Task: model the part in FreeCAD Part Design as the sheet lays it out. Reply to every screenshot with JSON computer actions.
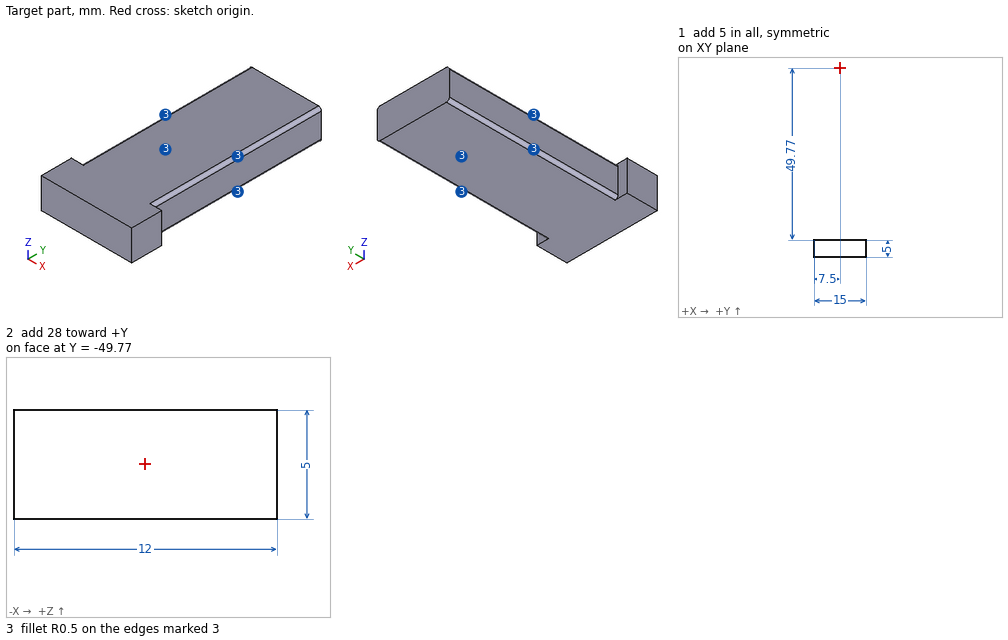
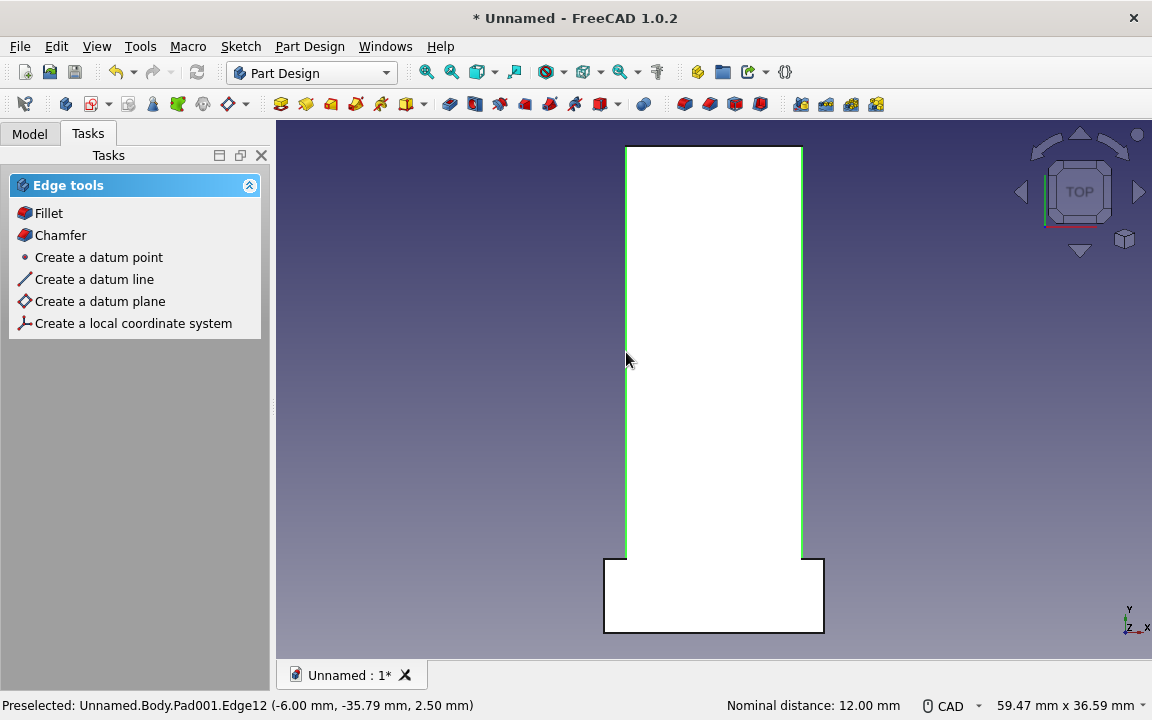
{"action": "left_click", "coordinate": [427, 72]}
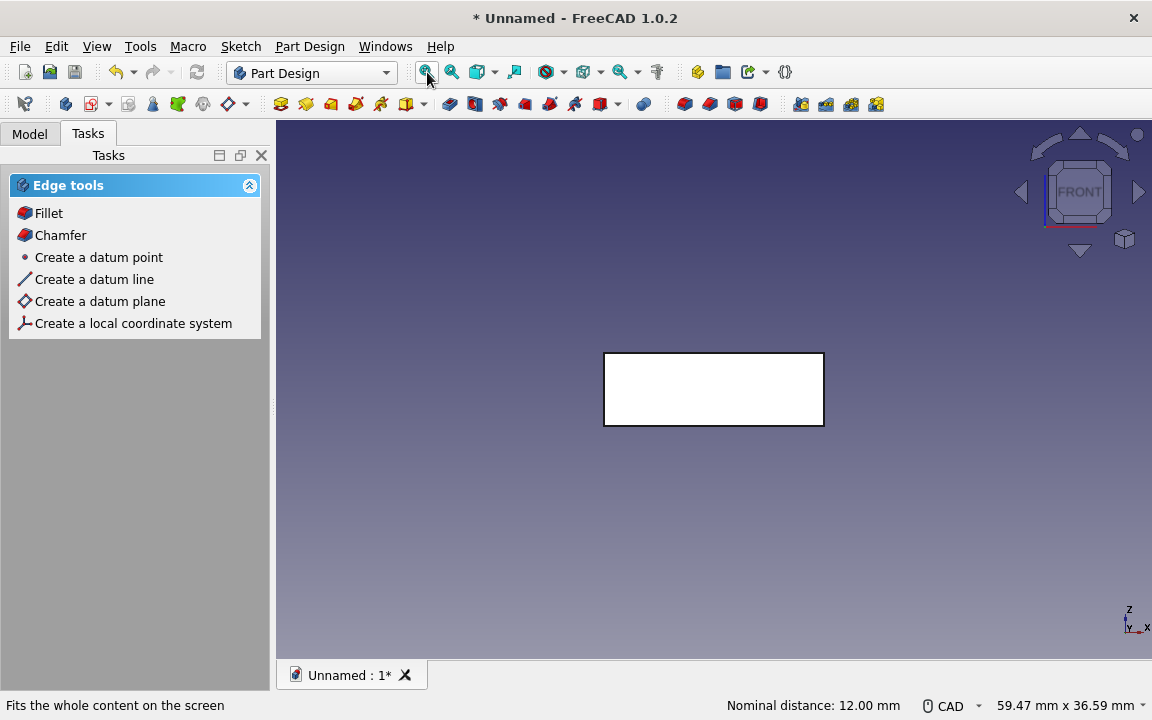
{"action": "key", "text": "3"}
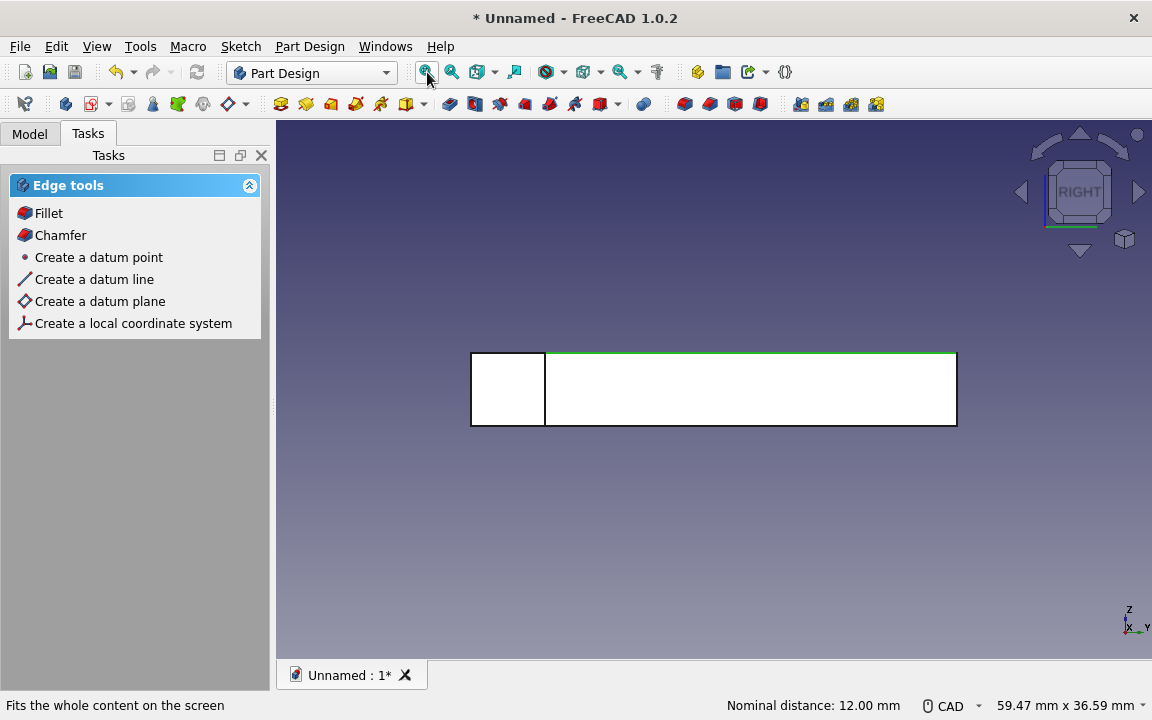
{"action": "left_click", "coordinate": [751, 425], "text": "ctrl"}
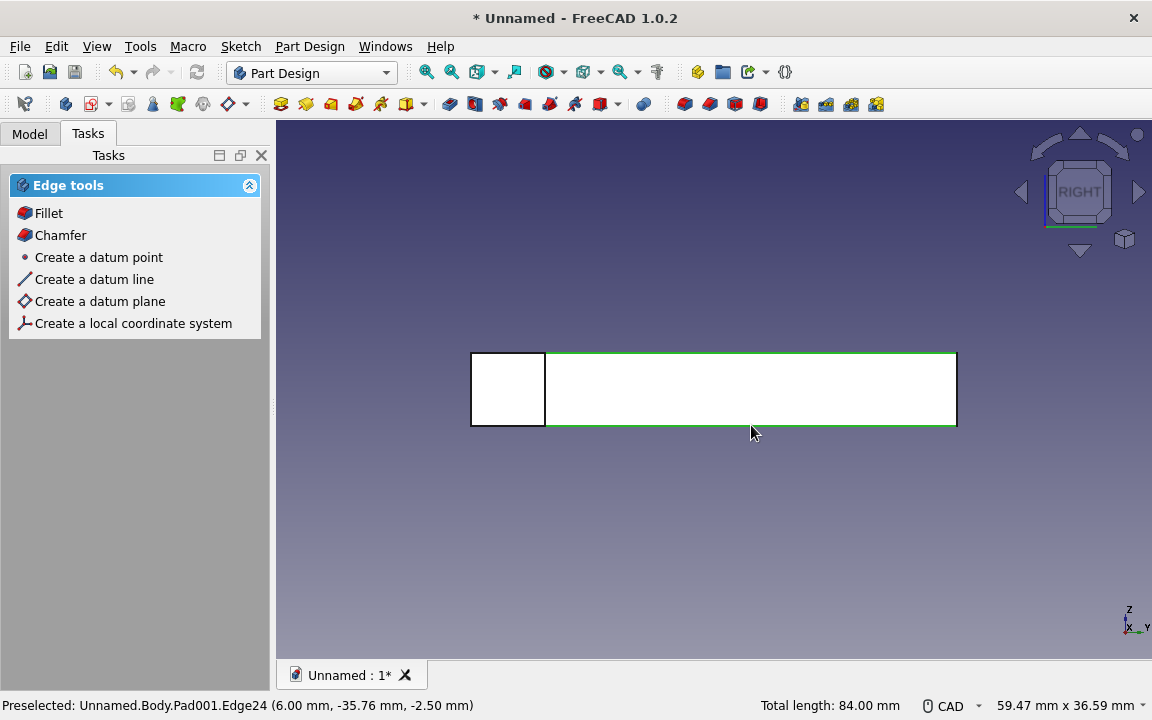
{"action": "key", "text": "5"}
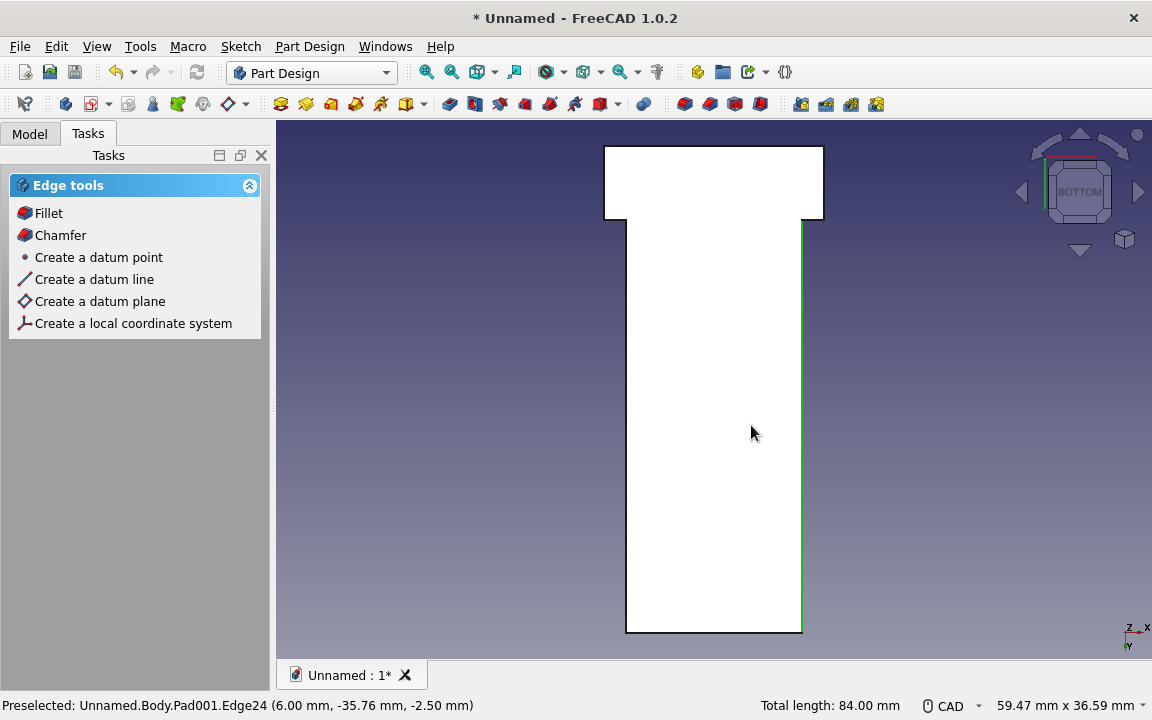
{"action": "left_click", "coordinate": [626, 425], "text": "ctrl"}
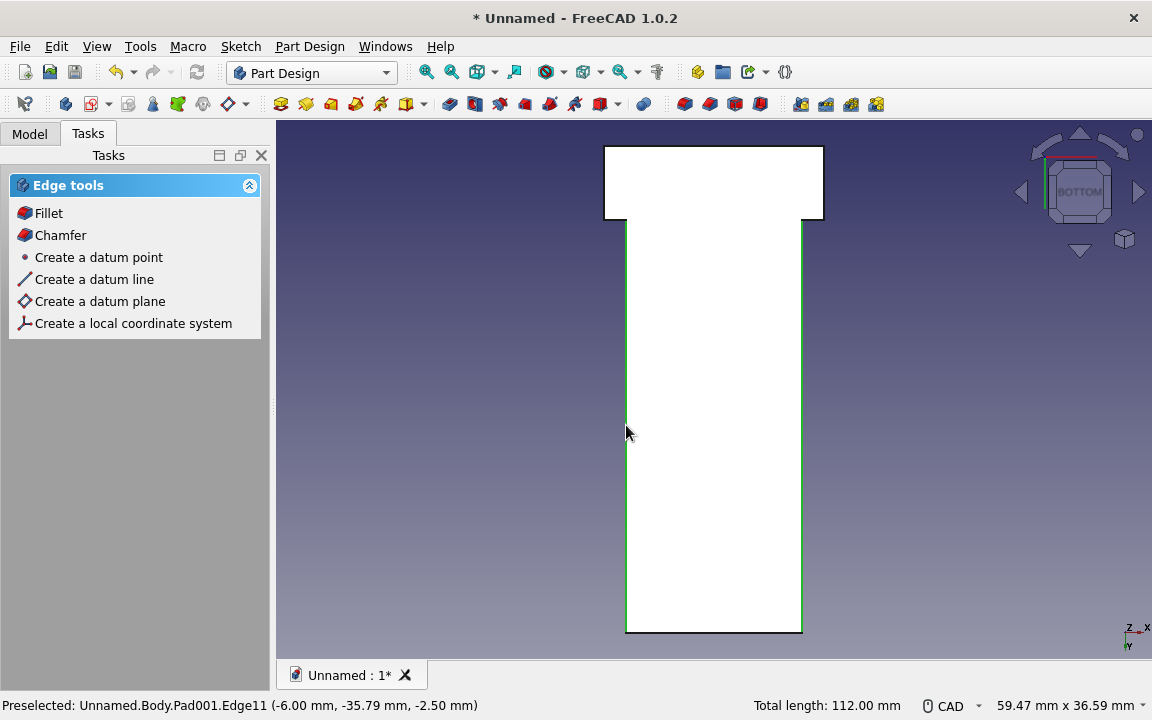
{"action": "left_click", "coordinate": [685, 104]}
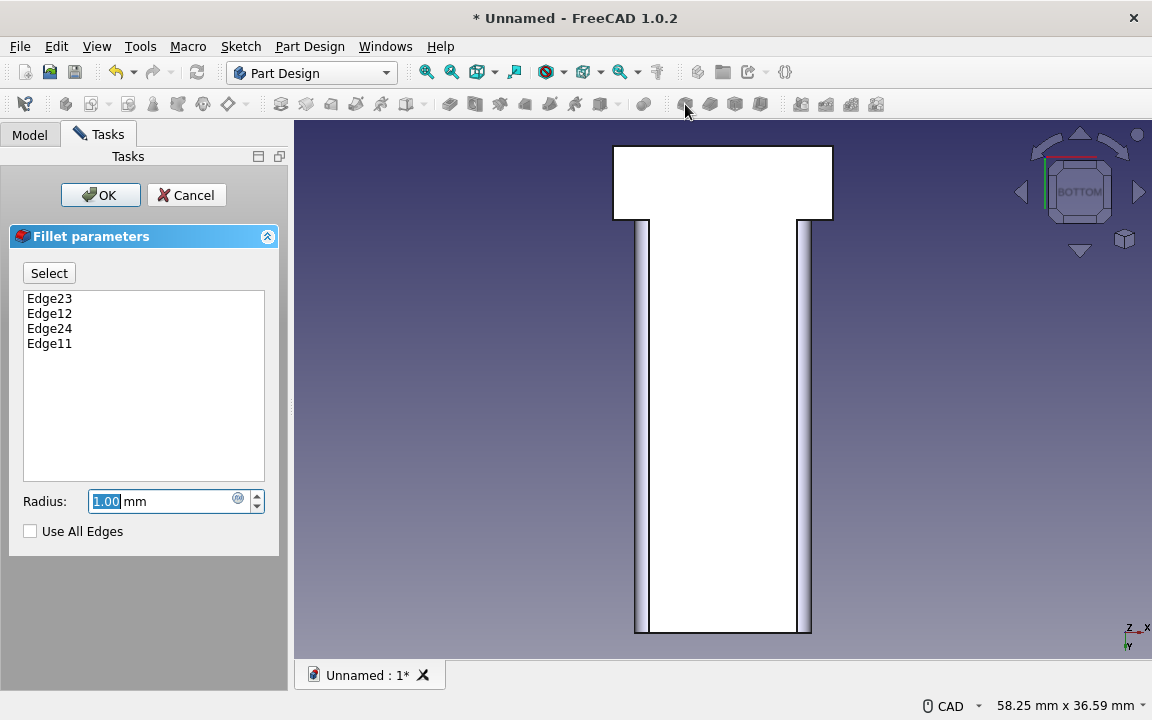
{"action": "type", "text": "0.5"}
{"action": "key", "text": "Tab"}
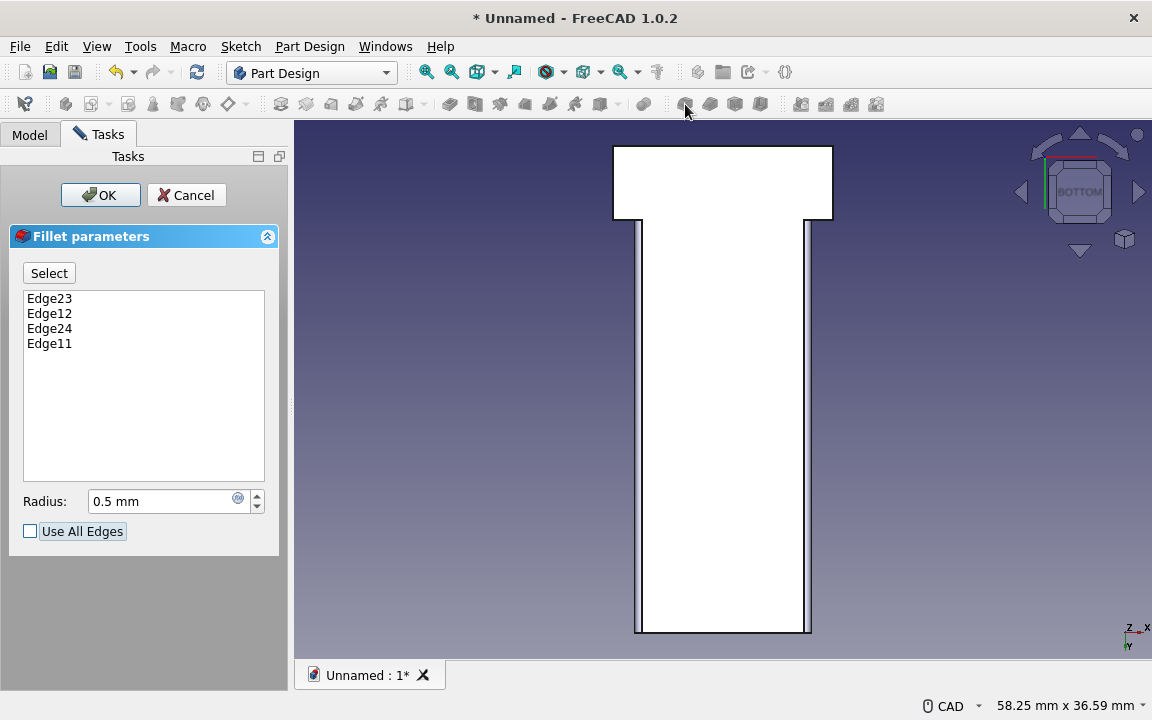
{"action": "left_click", "coordinate": [101, 195]}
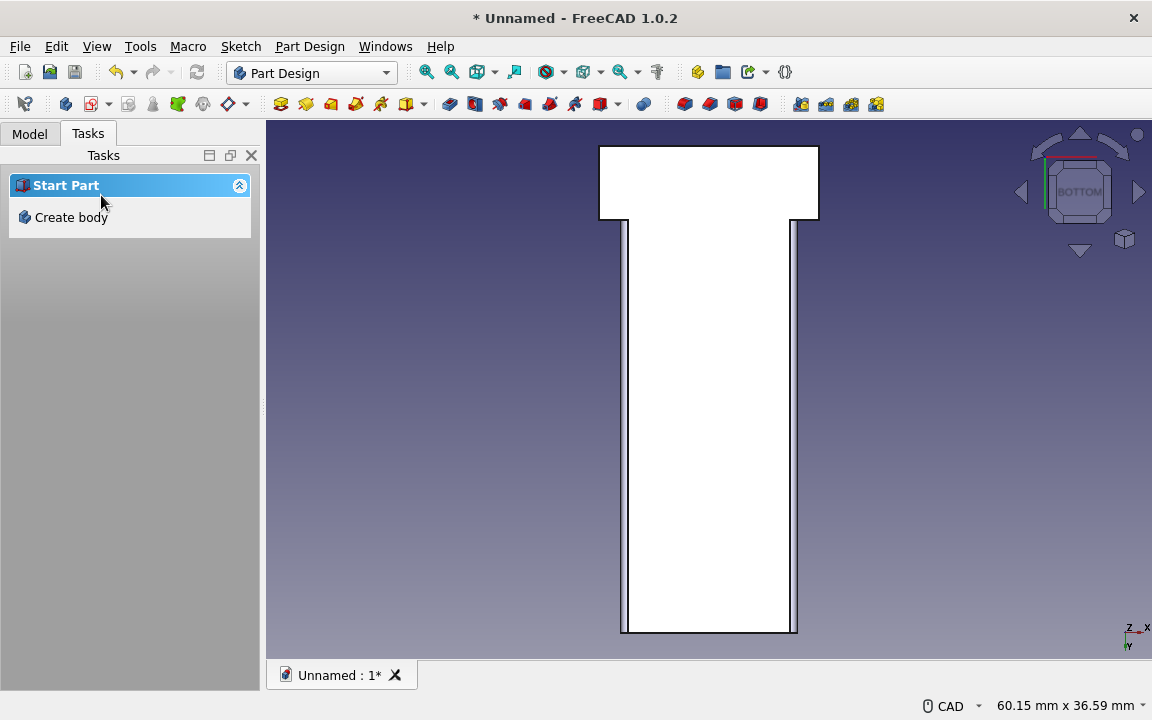
{"action": "key", "text": "0"}